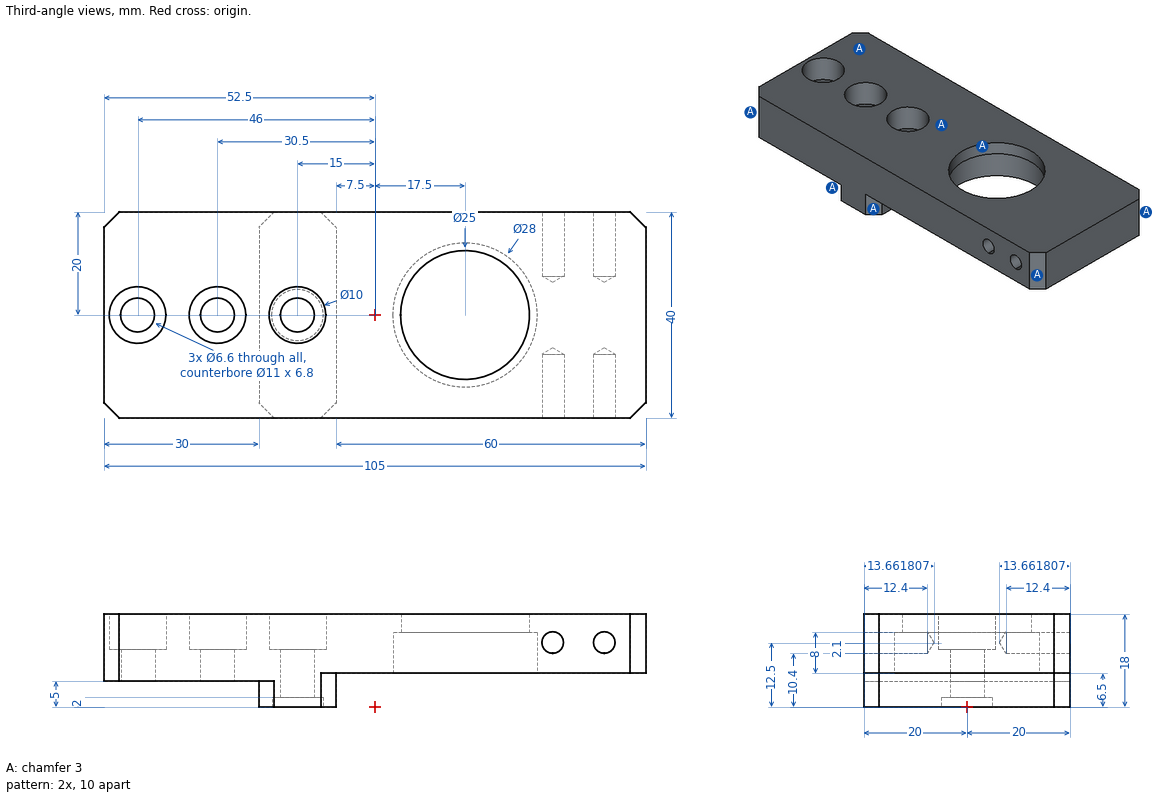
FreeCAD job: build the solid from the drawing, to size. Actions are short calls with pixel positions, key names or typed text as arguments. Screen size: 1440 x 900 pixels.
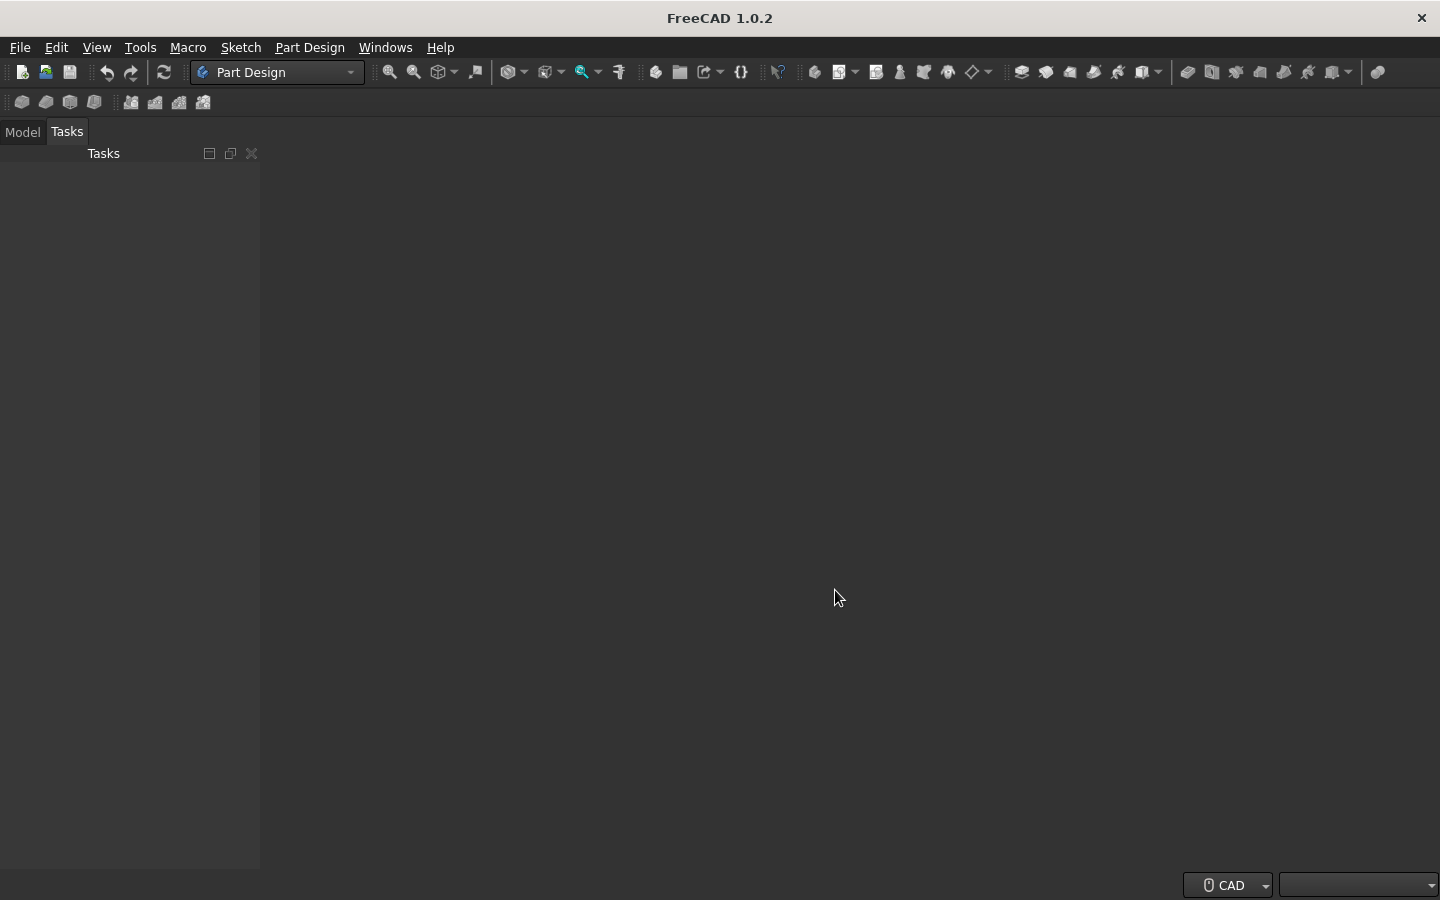
click(22, 72)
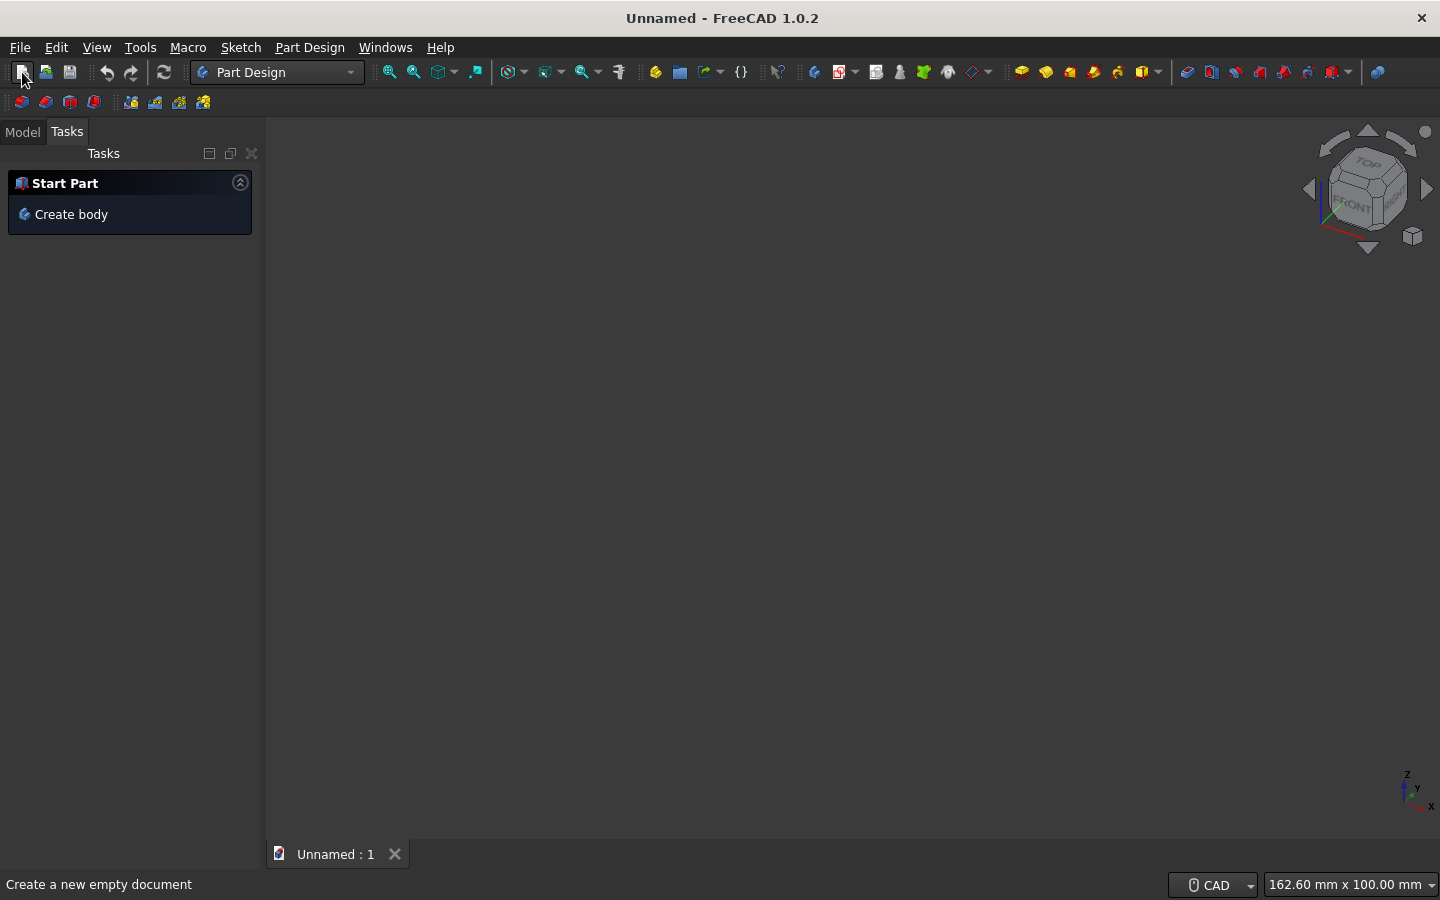
click(840, 72)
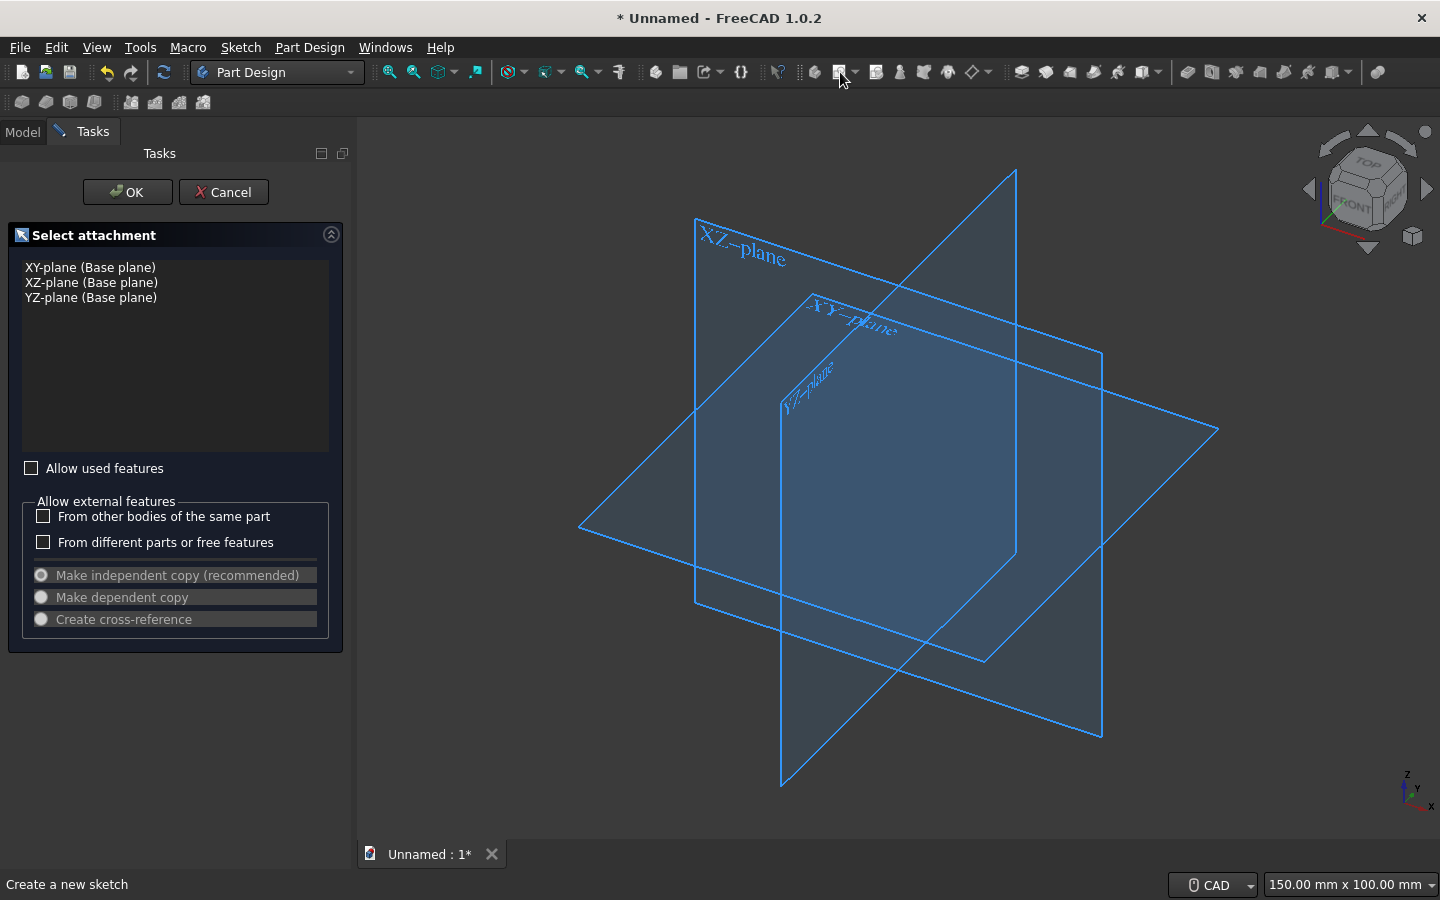
click(82, 268)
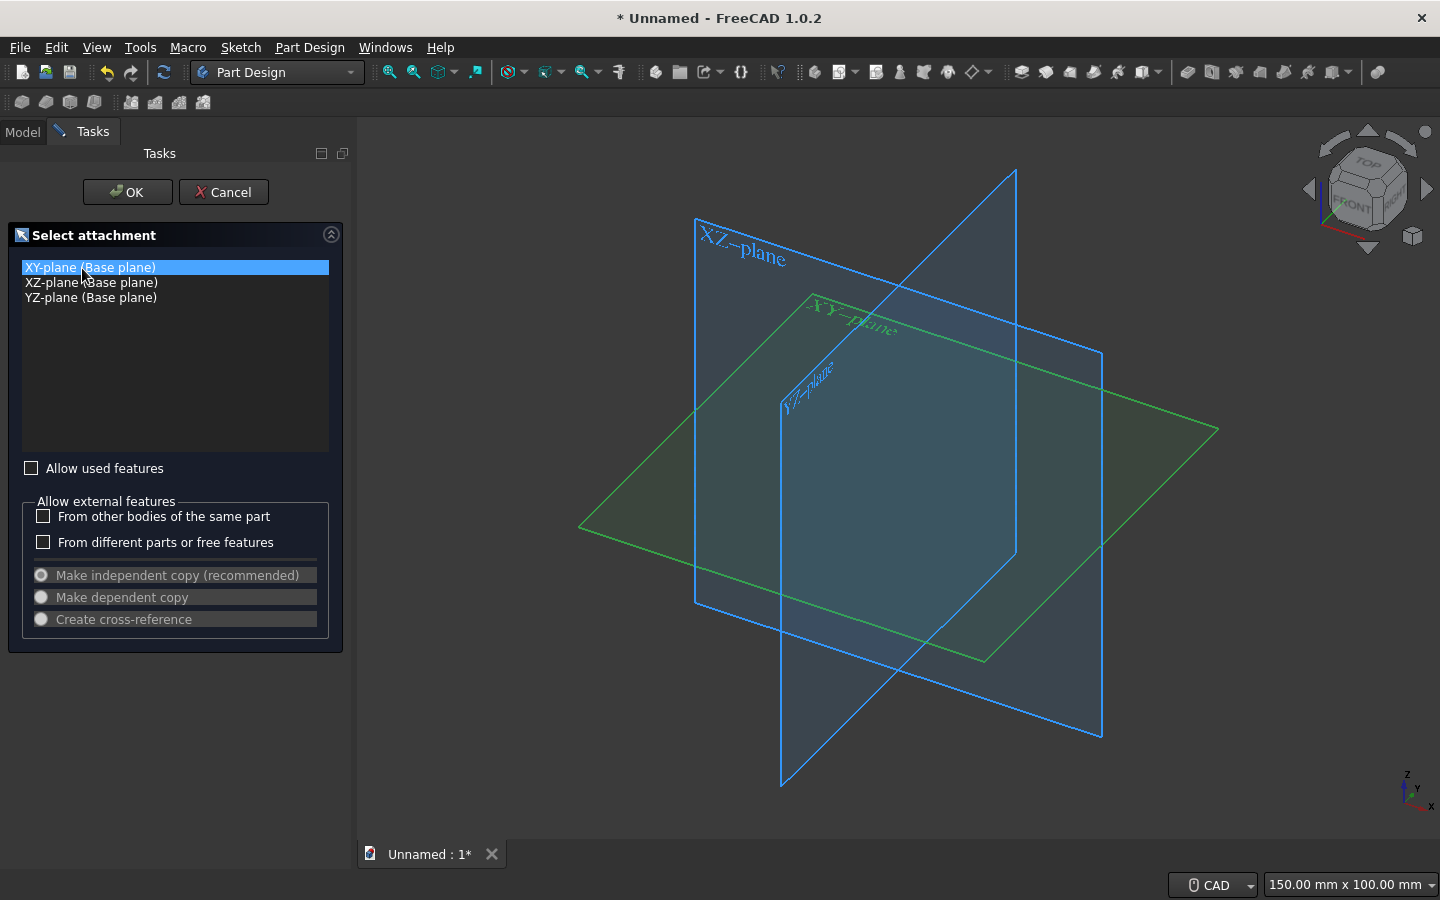
click(128, 192)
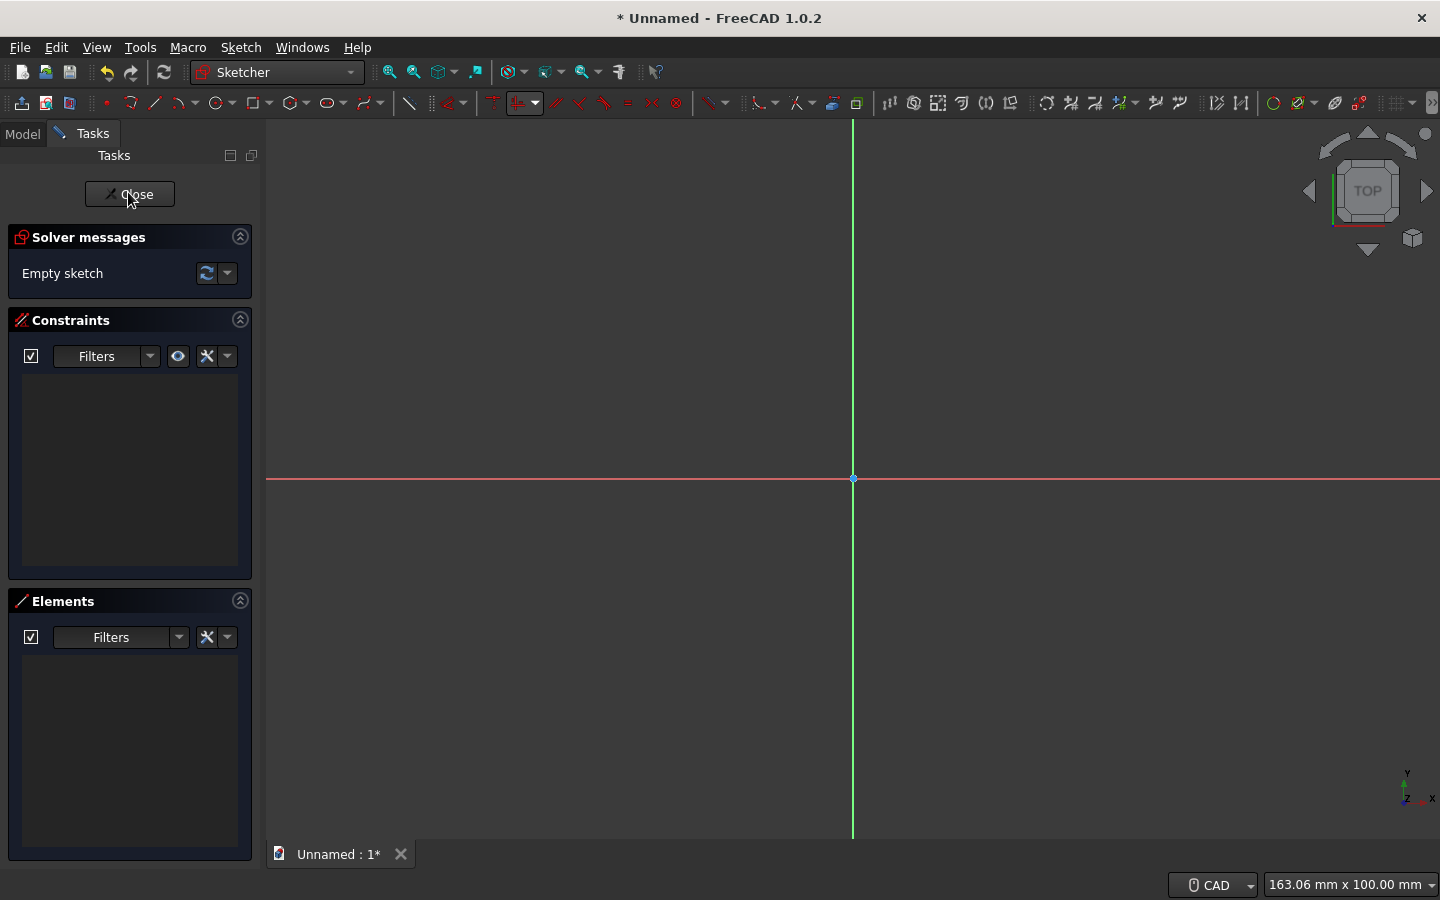
click(272, 104)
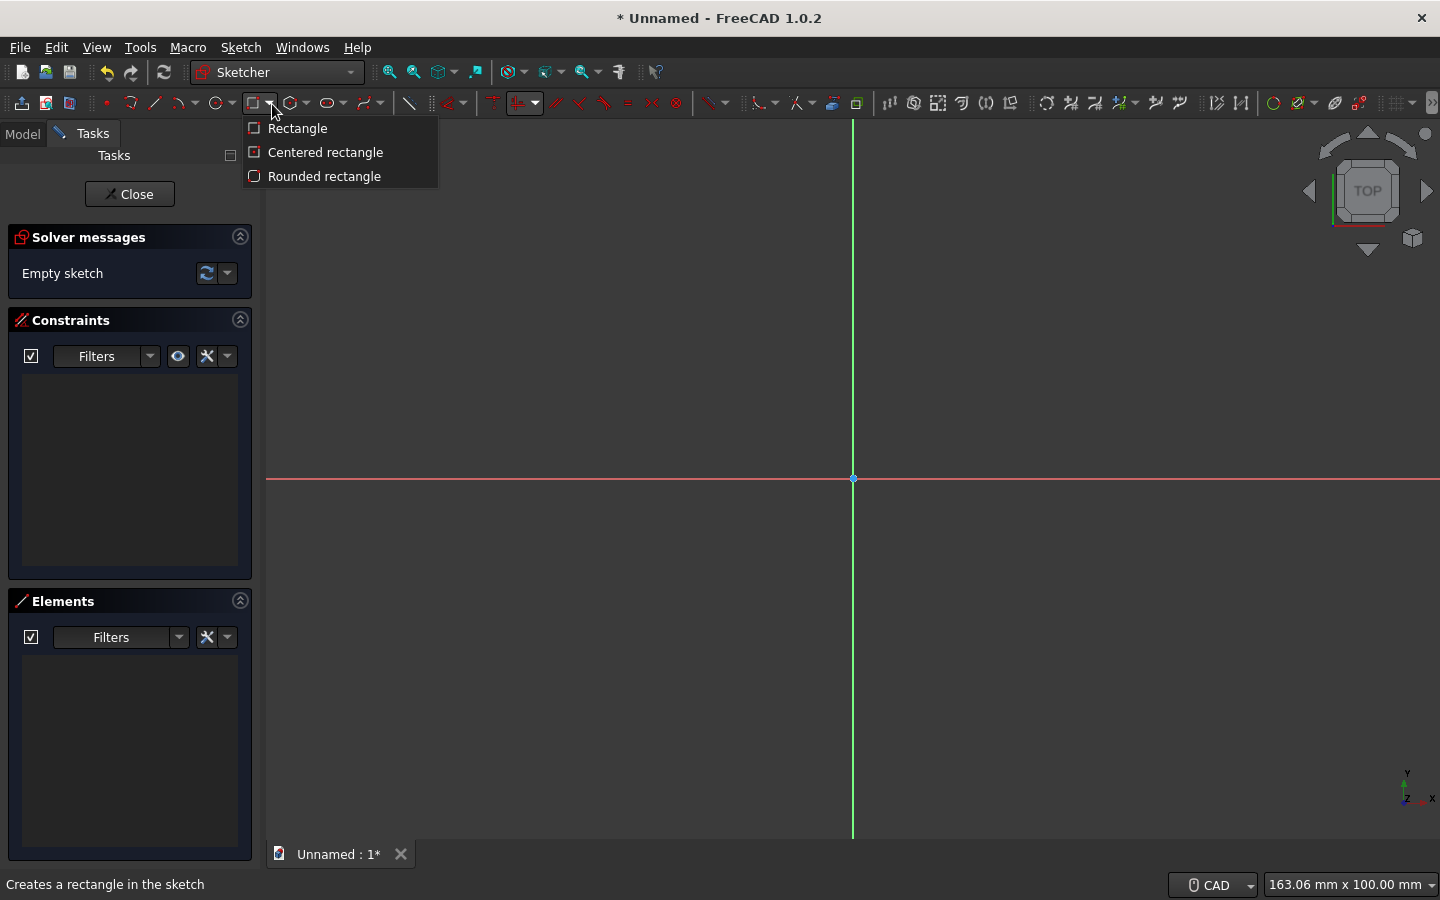
click(340, 152)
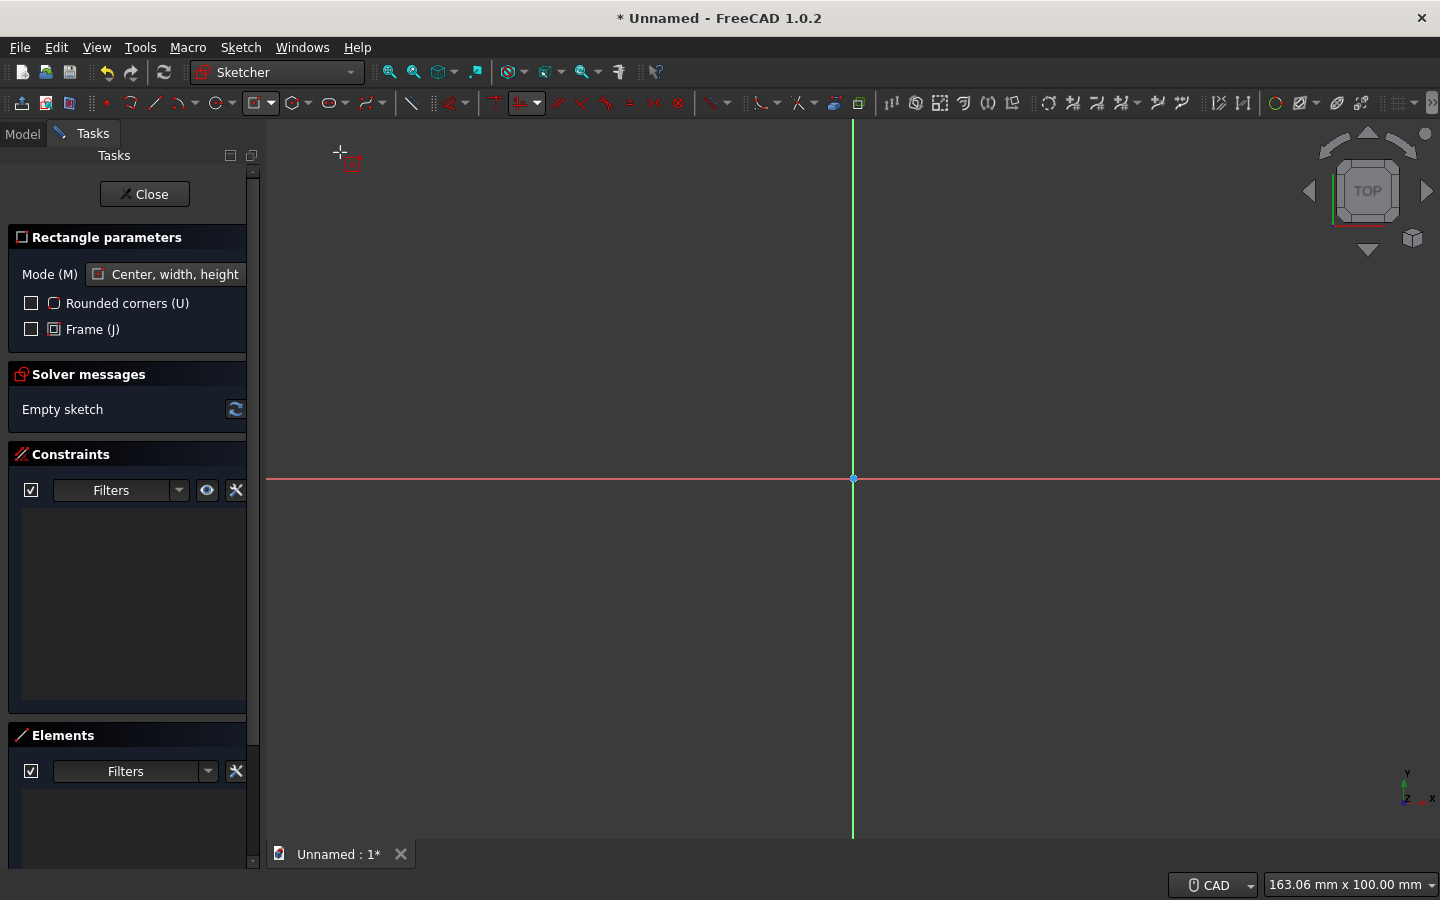
click(853, 479)
click(1231, 335)
key(Escape)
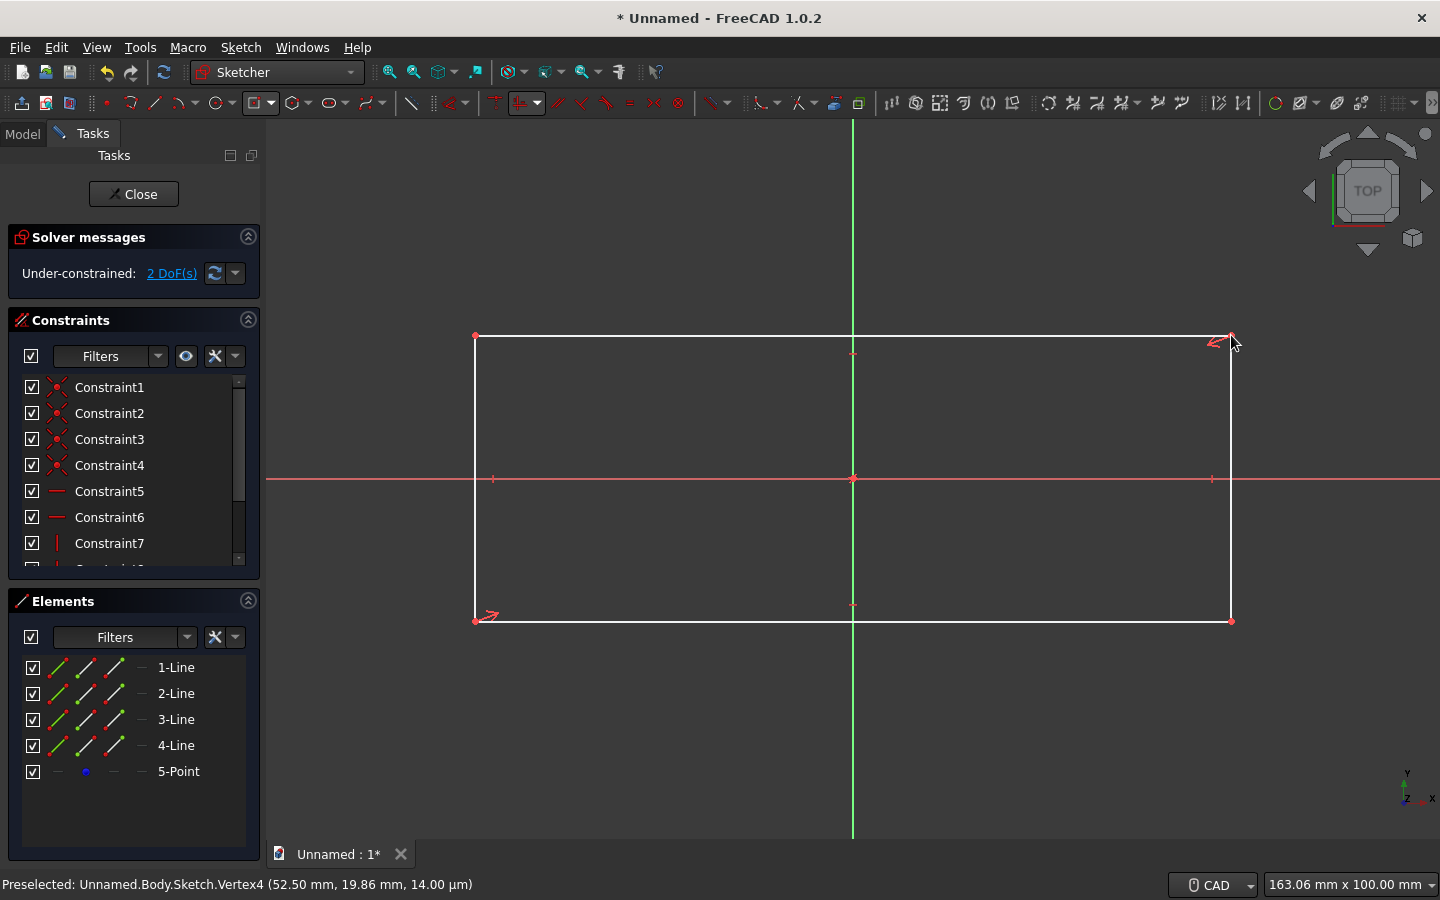
click(1231, 536)